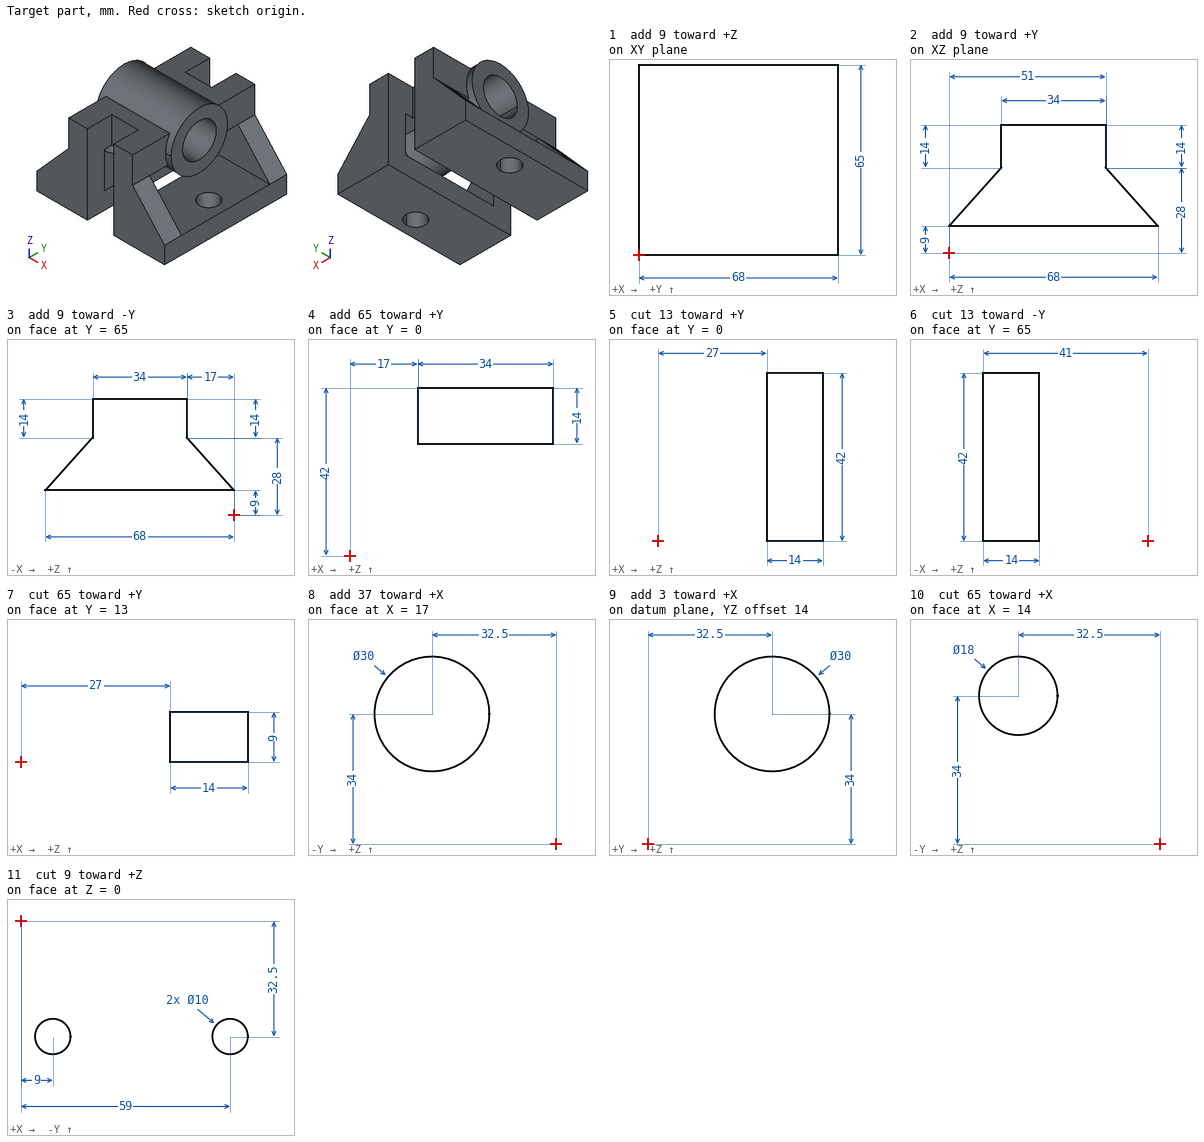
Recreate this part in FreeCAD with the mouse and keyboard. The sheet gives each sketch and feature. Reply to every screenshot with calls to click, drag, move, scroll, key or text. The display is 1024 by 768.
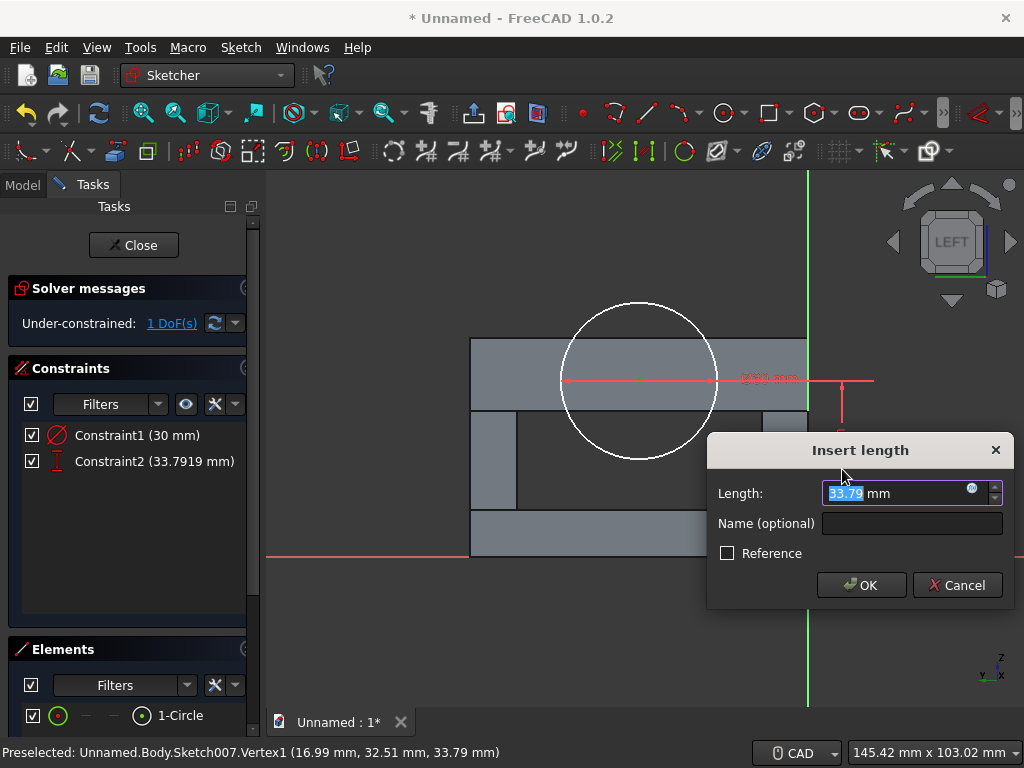
text(34)
key(Return)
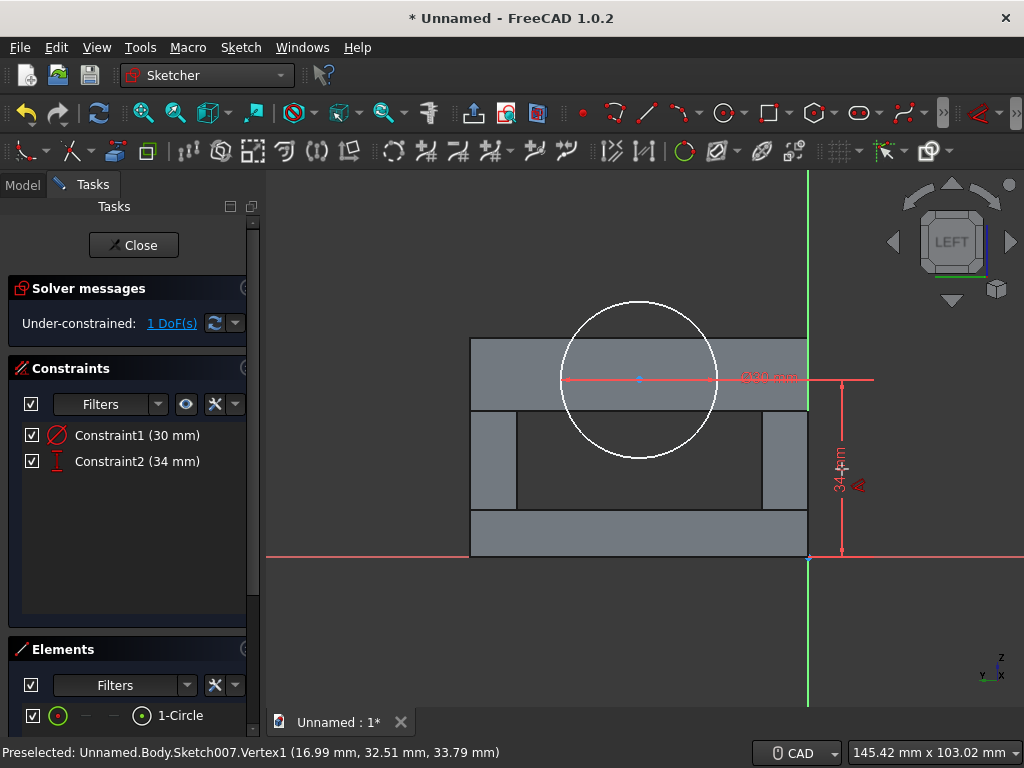
click(639, 380)
click(724, 591)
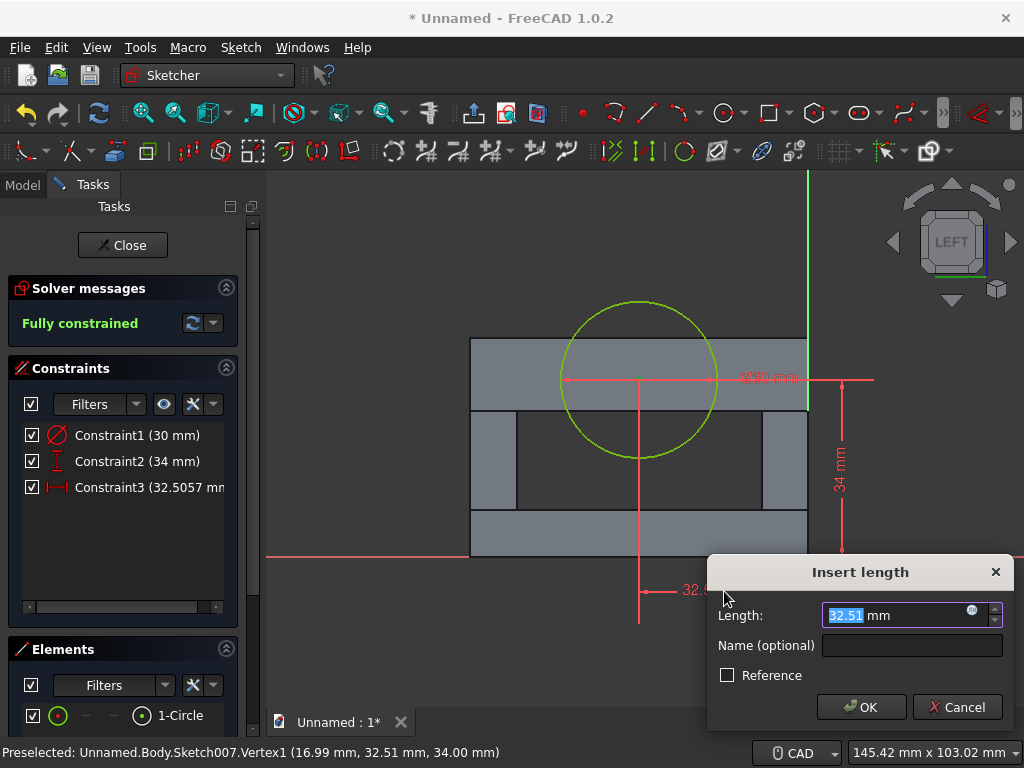
text(32.5)
key(Return)
key(Escape)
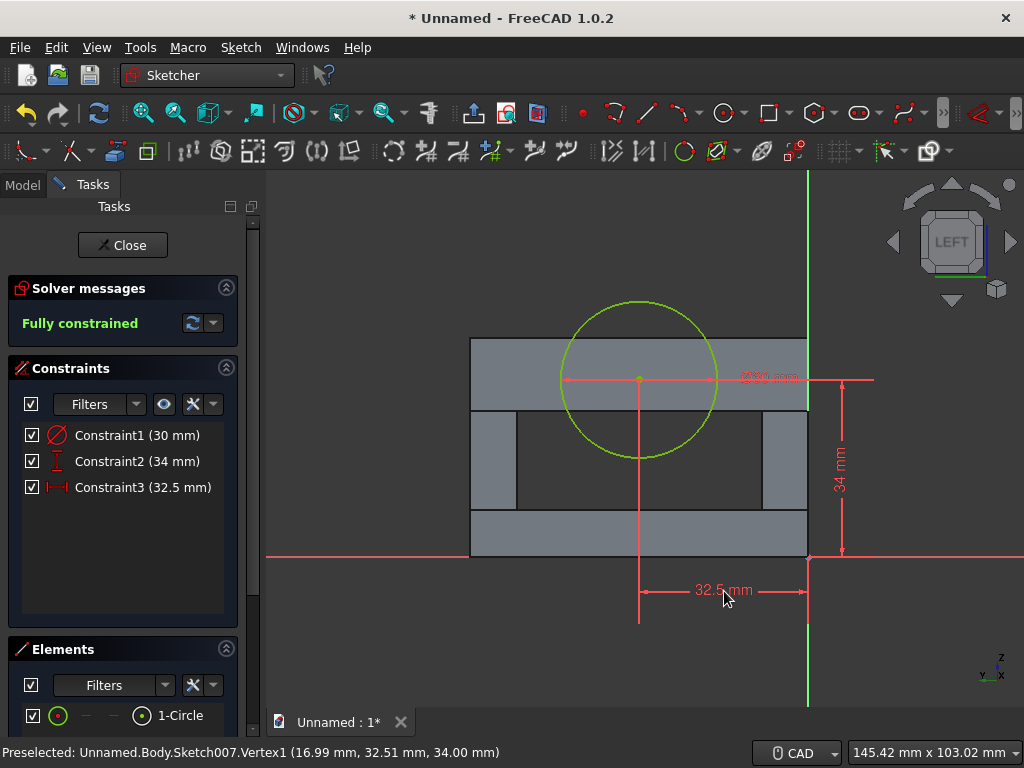
click(123, 245)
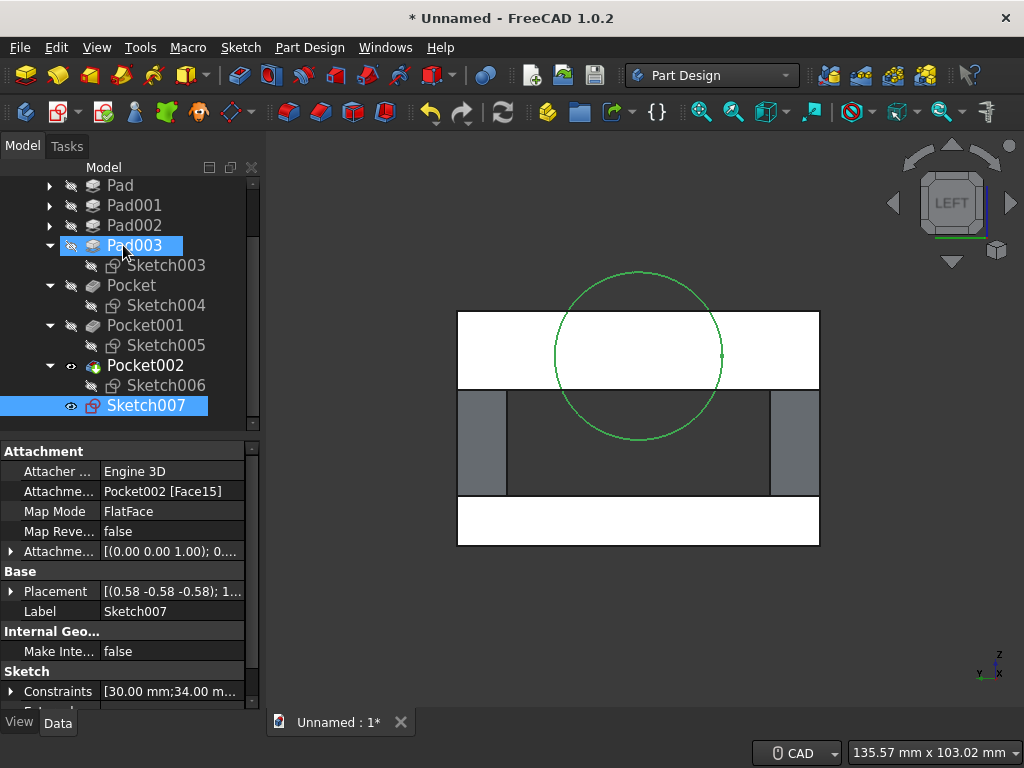
click(26, 76)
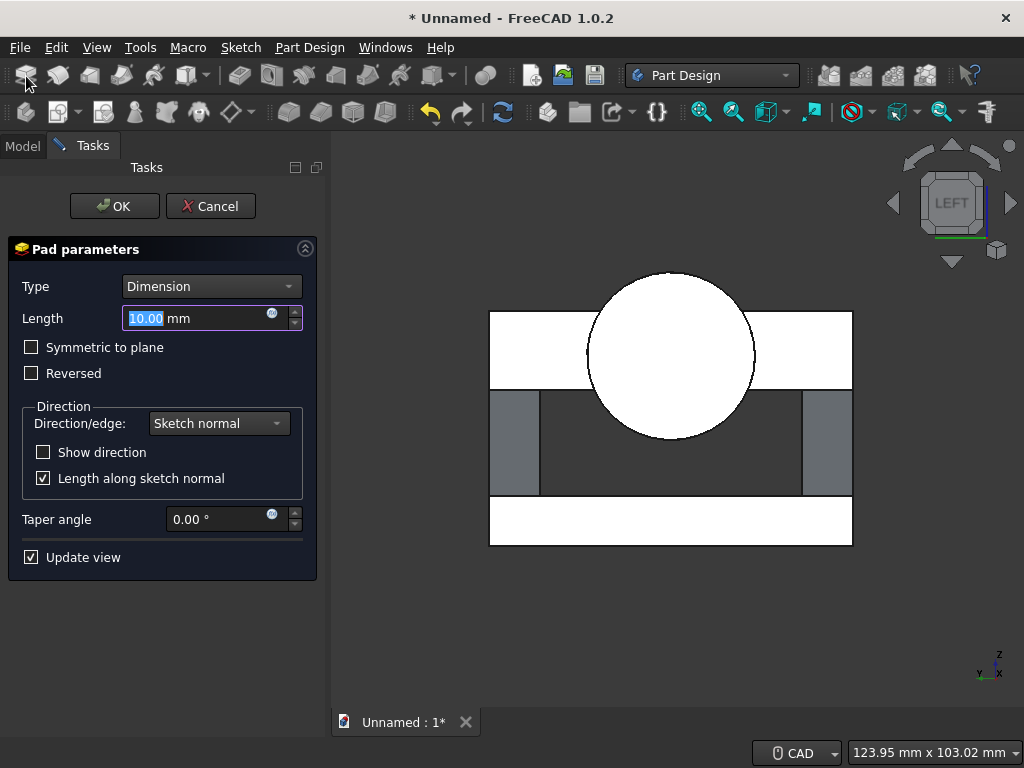
text(37)
key(Tab)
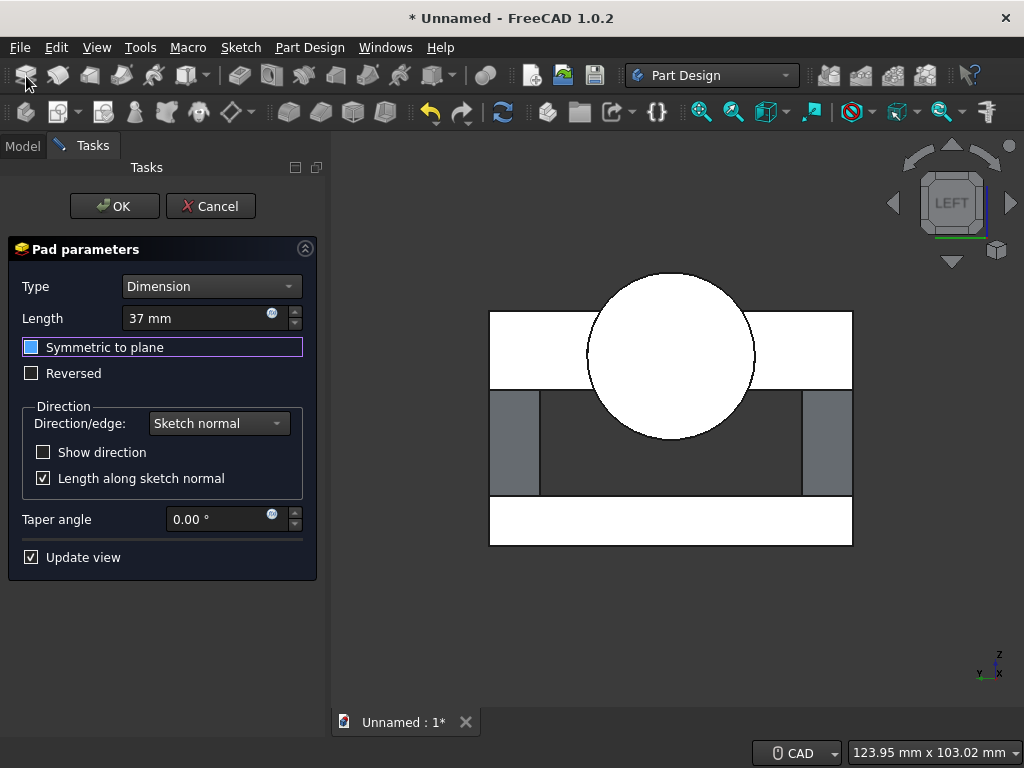
click(30, 373)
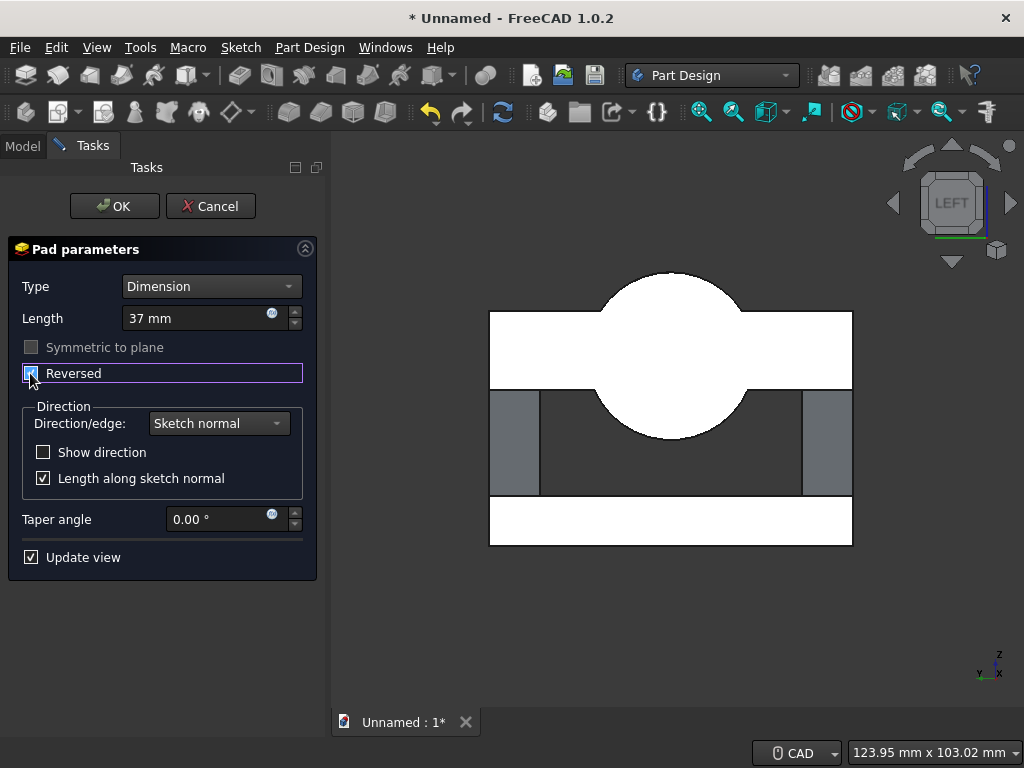
click(115, 206)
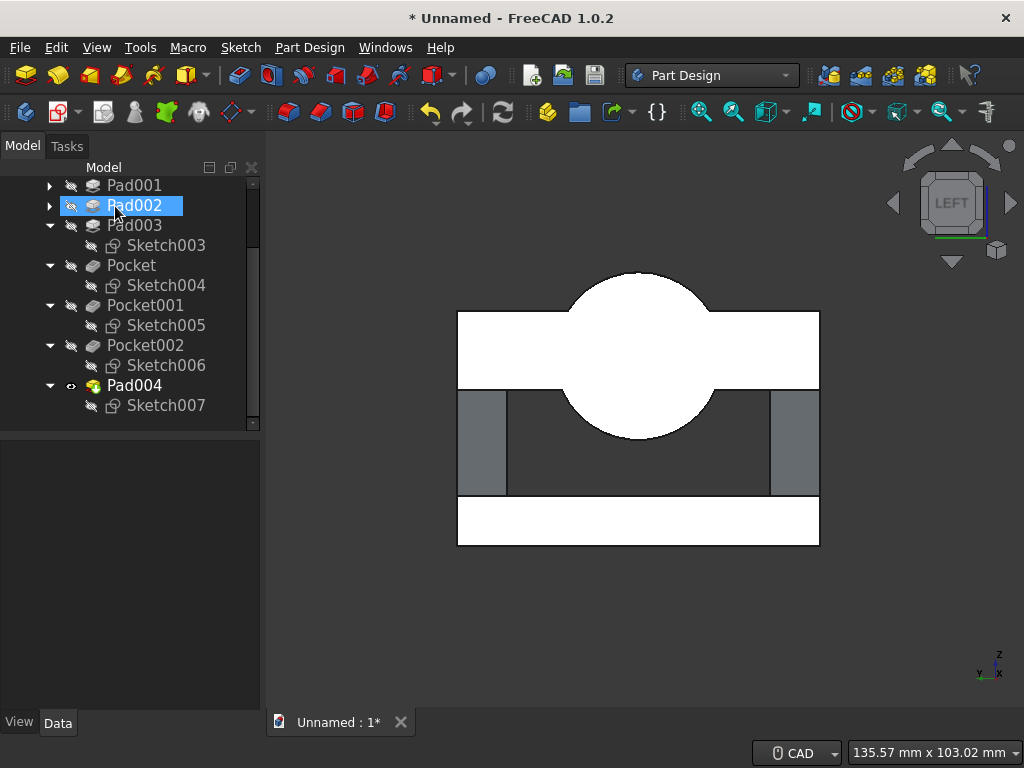
scroll(140, 301, down, 3)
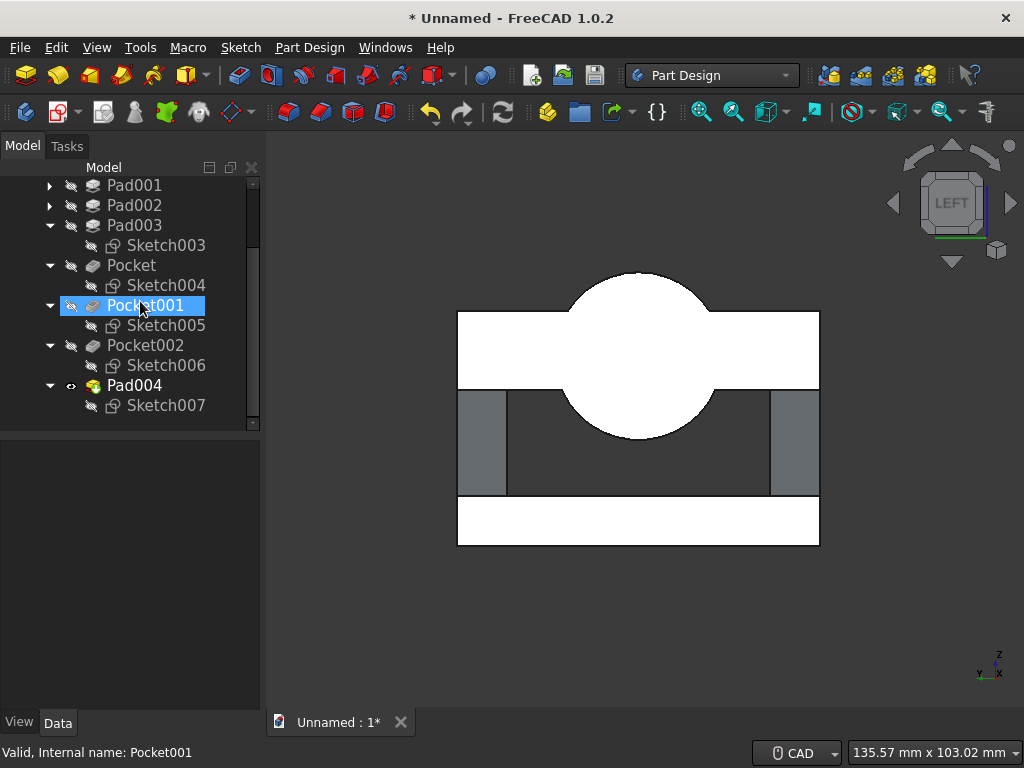
scroll(140, 301, up, 15)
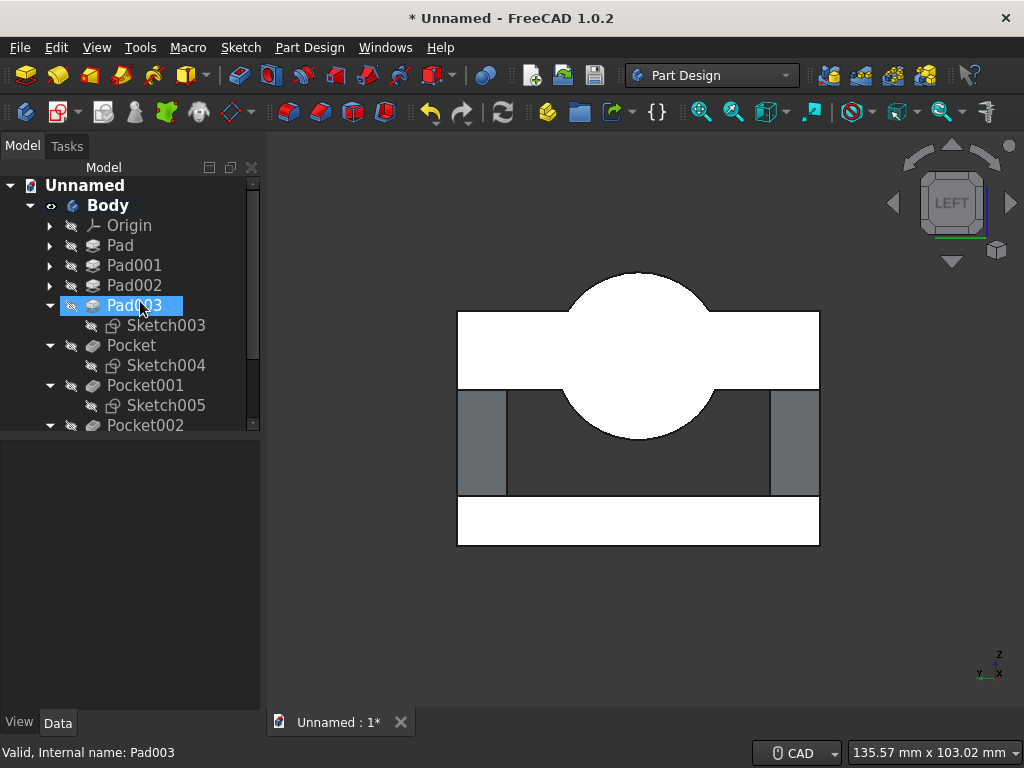
click(50, 226)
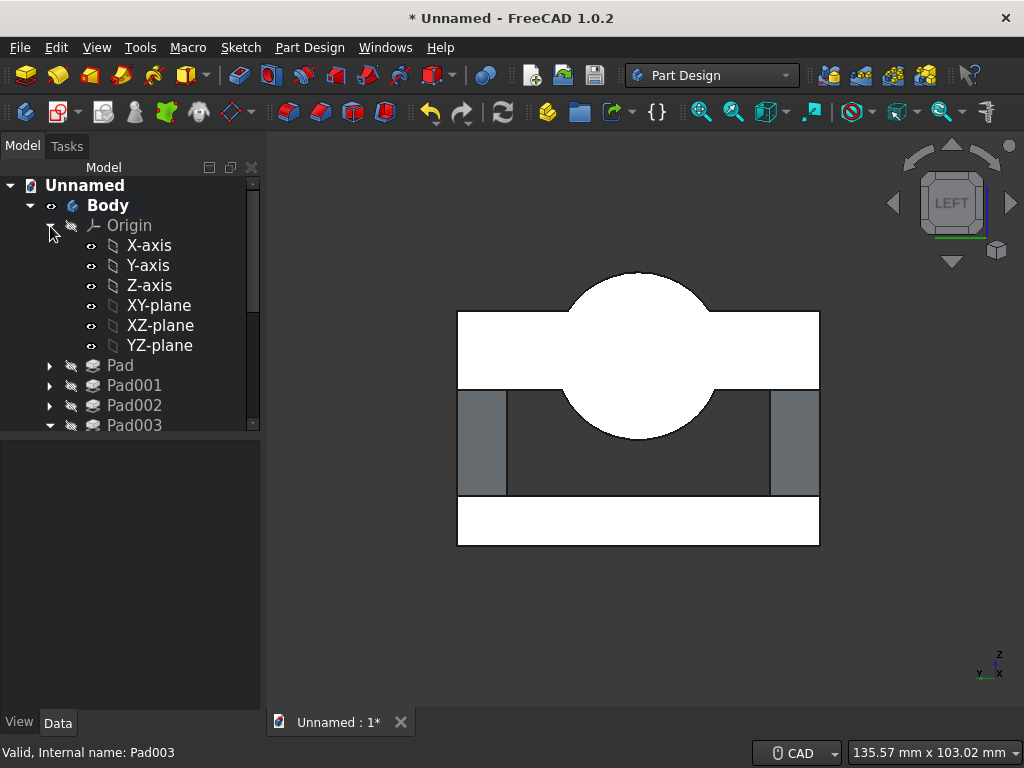
click(136, 346)